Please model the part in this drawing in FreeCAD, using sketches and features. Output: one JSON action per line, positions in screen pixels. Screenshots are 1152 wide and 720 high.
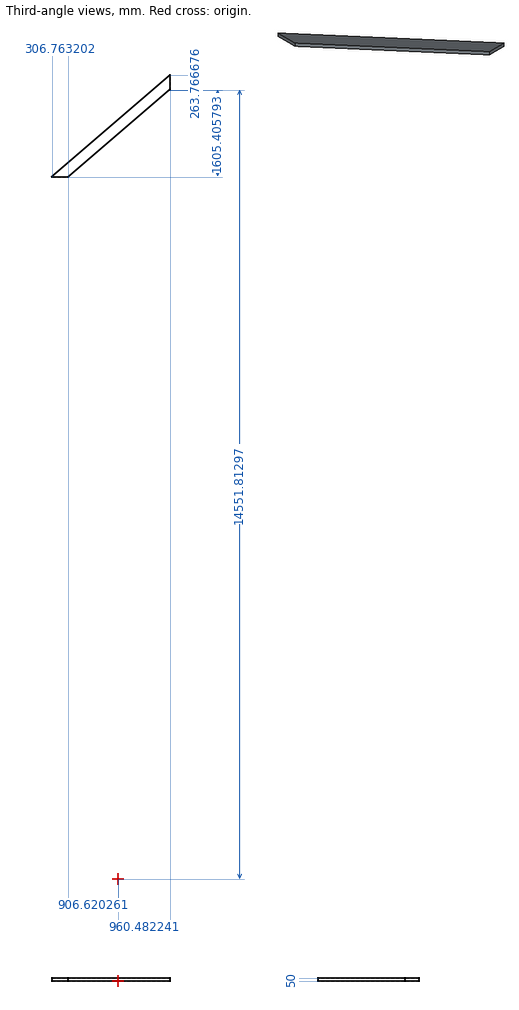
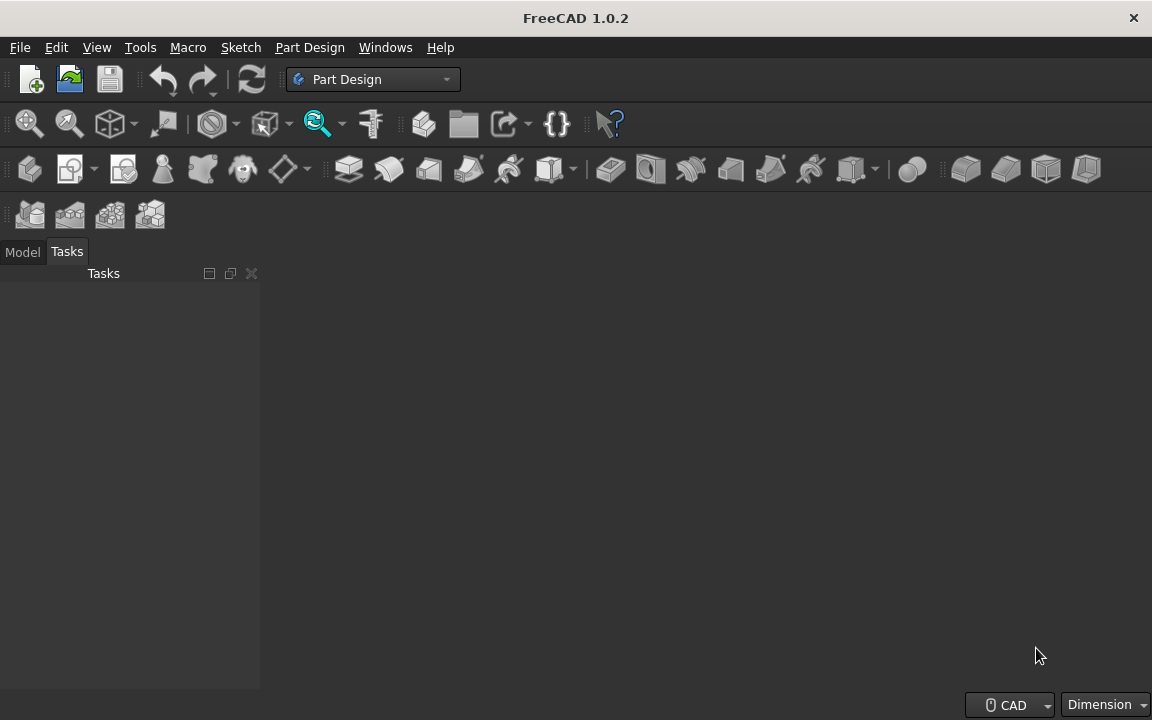
{"action": "key", "text": "ctrl+n"}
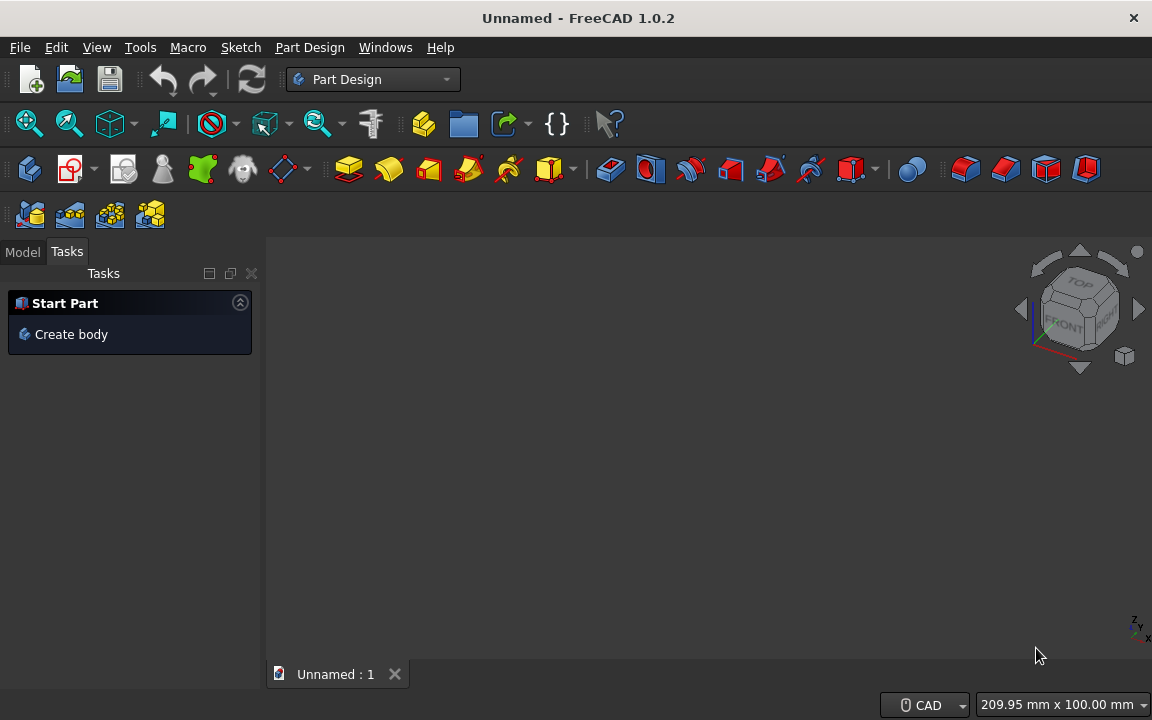
{"action": "left_click", "coordinate": [70, 170]}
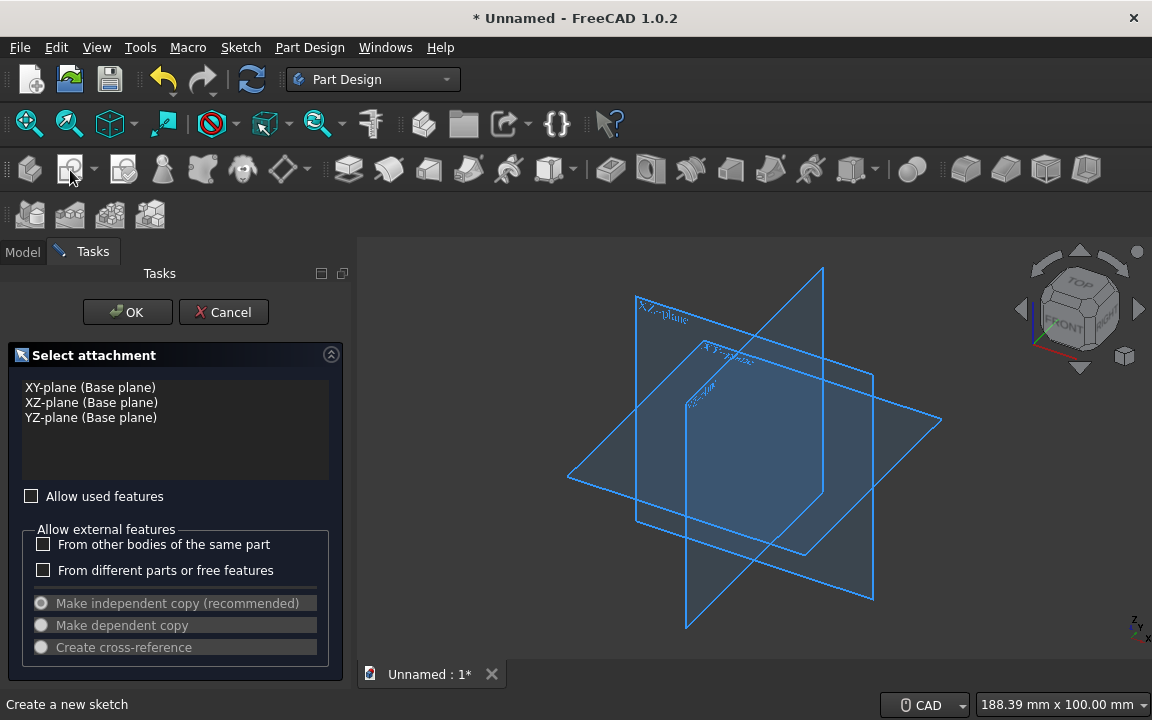
{"action": "left_click", "coordinate": [82, 388]}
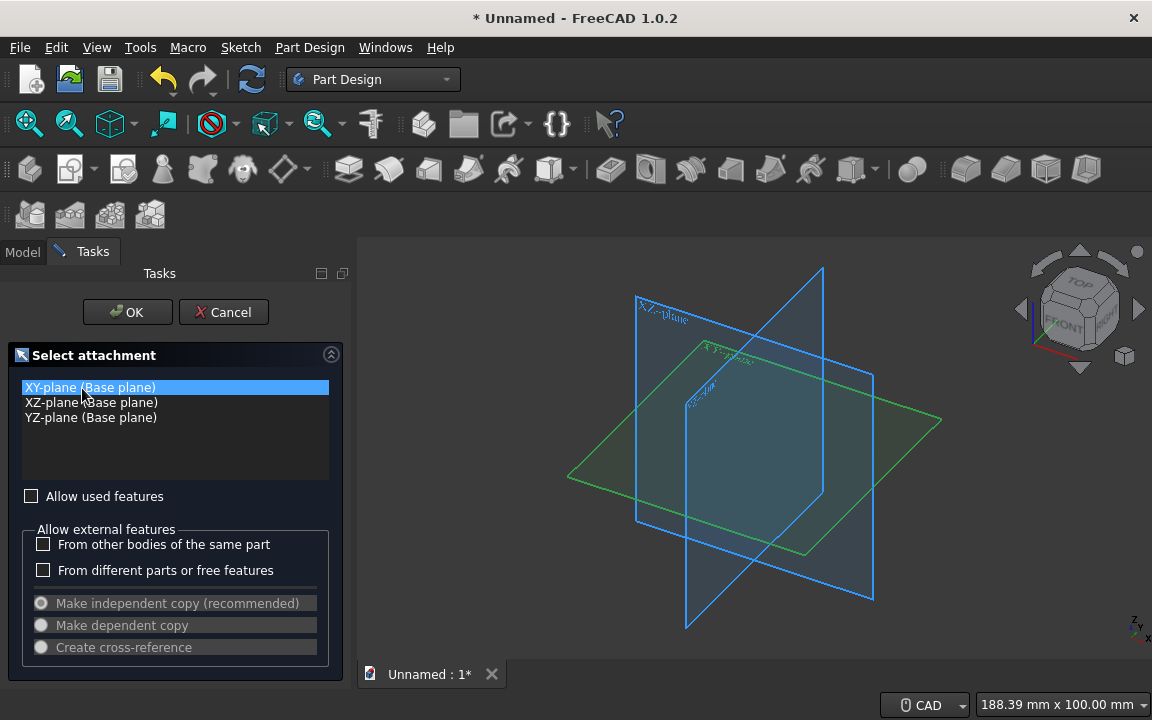
{"action": "left_click", "coordinate": [128, 312]}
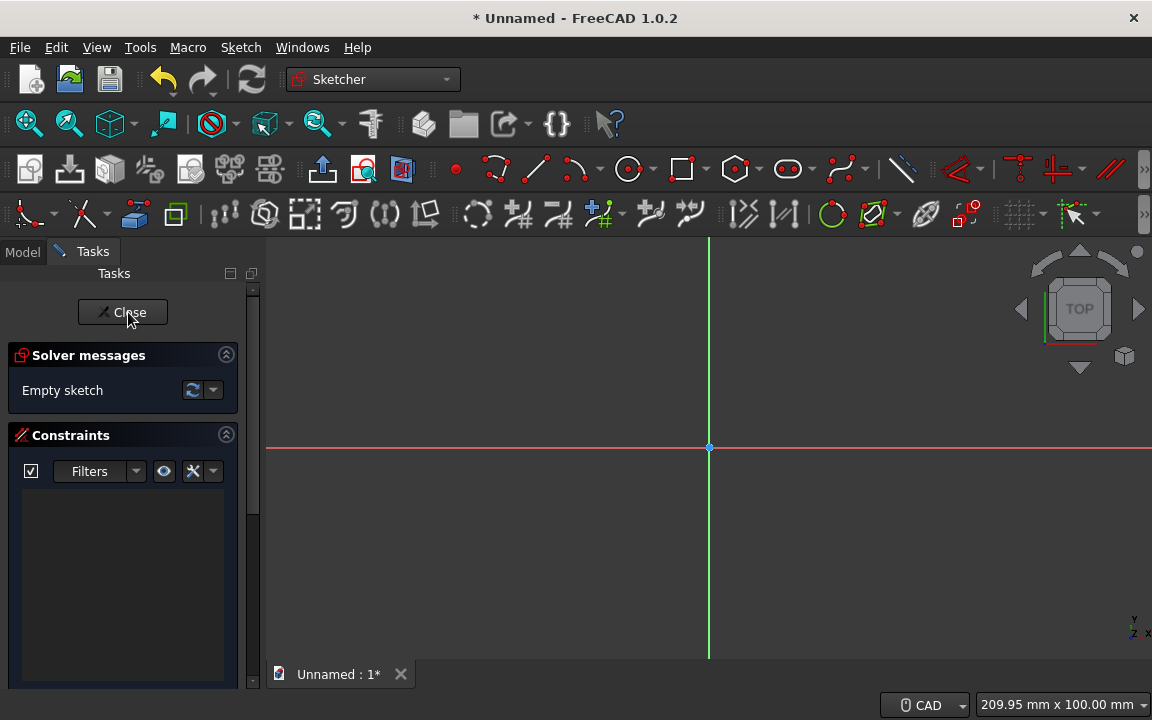
{"action": "scroll", "coordinate": [640, 448], "scroll_direction": "down", "scroll_amount": 15}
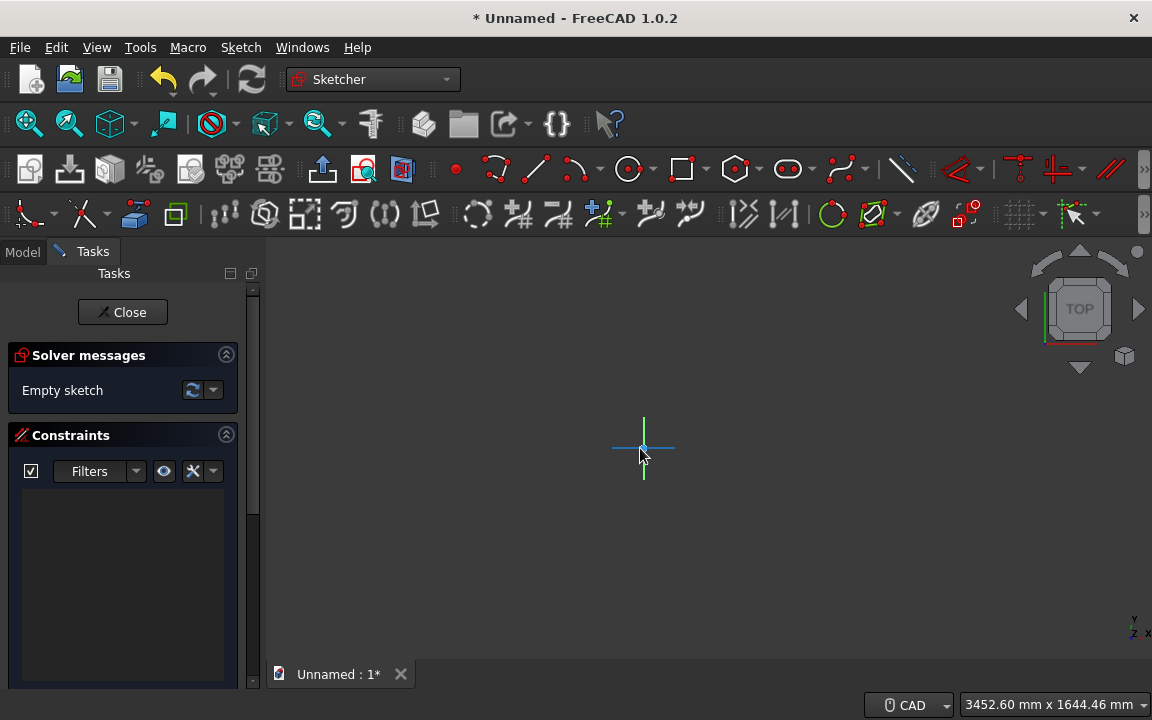
{"action": "scroll", "coordinate": [640, 448], "scroll_direction": "down", "scroll_amount": 5}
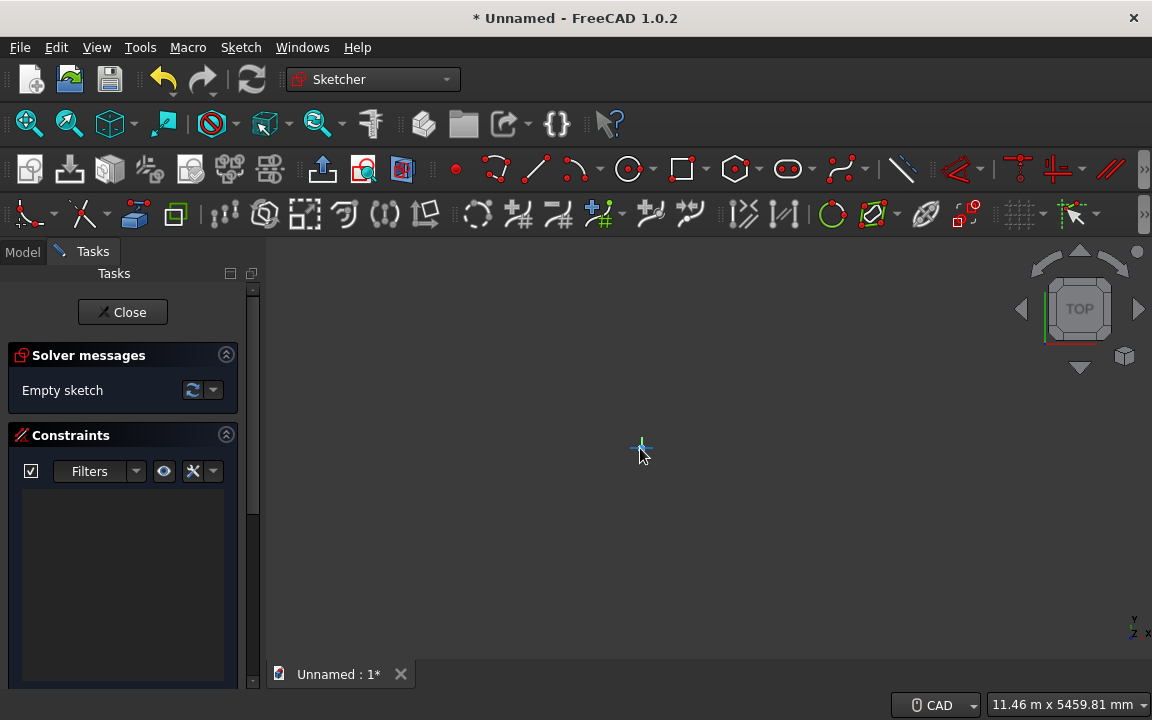
{"action": "scroll", "coordinate": [640, 448], "scroll_direction": "down", "scroll_amount": 5}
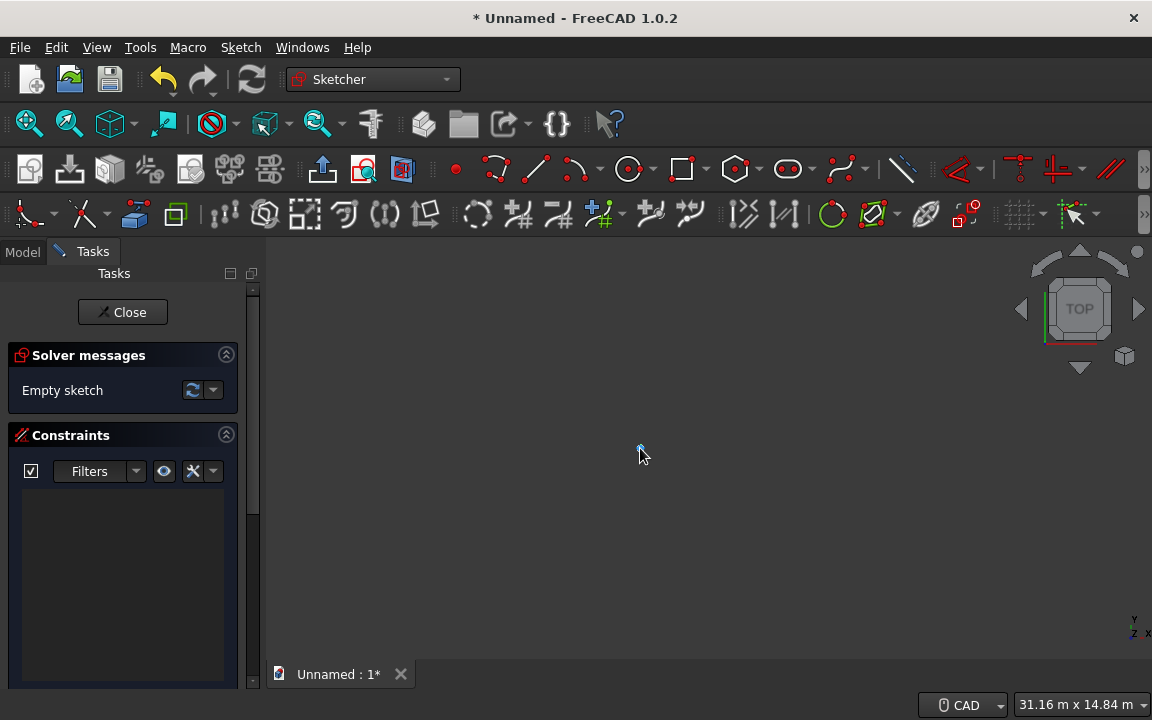
{"action": "scroll", "coordinate": [640, 448], "scroll_direction": "down", "scroll_amount": 5}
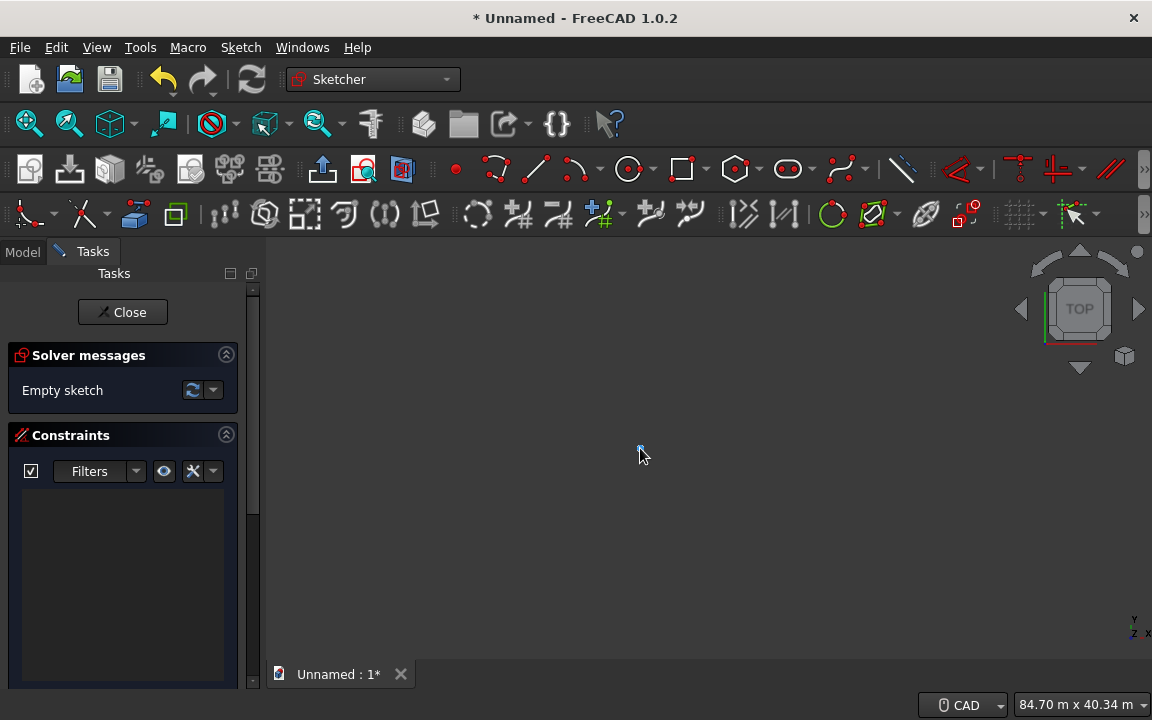
{"action": "scroll", "coordinate": [639, 292], "scroll_direction": "up", "scroll_amount": 13}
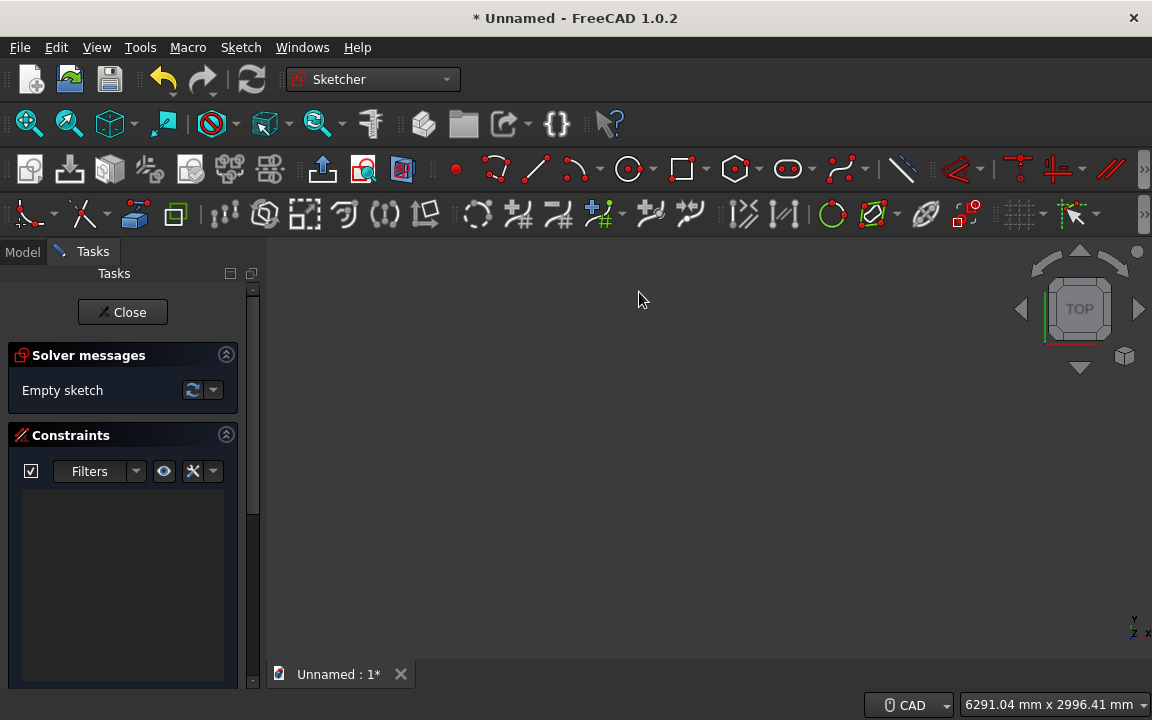
{"action": "key", "text": "g m"}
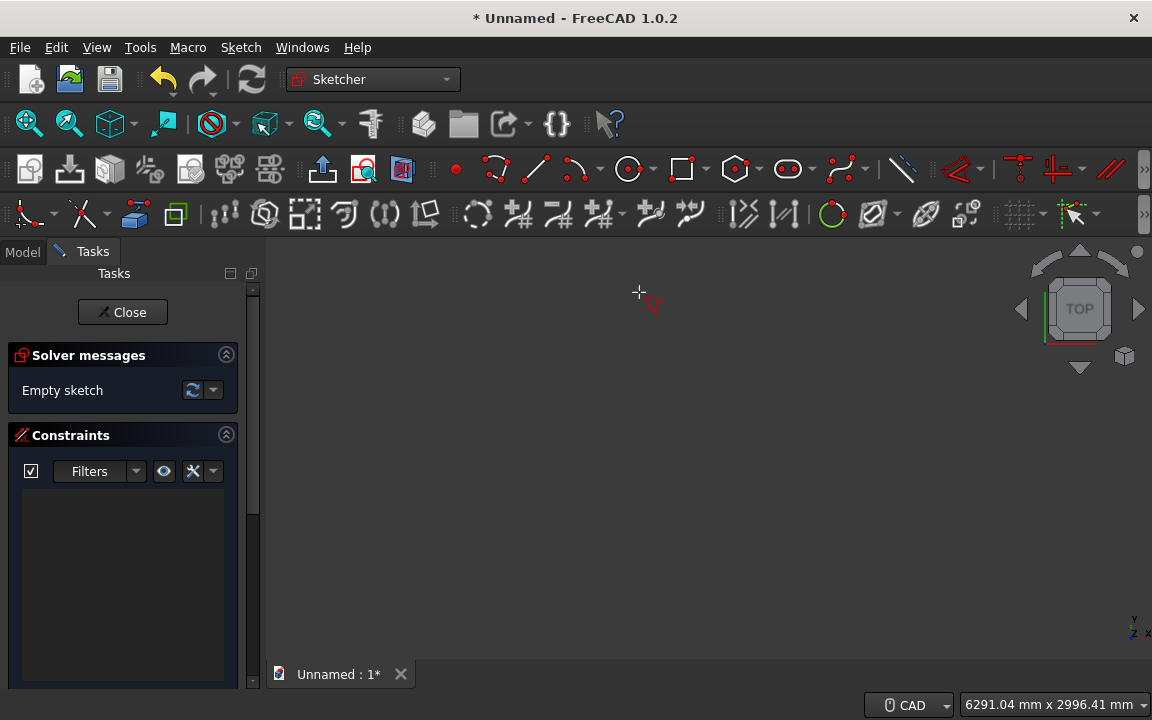
{"action": "left_click", "coordinate": [528, 574]}
{"action": "left_click", "coordinate": [790, 348]}
{"action": "left_click", "coordinate": [790, 311]}
{"action": "left_click", "coordinate": [484, 574]}
{"action": "left_click", "coordinate": [528, 575]}
{"action": "key", "text": "Escape"}
{"action": "key", "text": "Escape"}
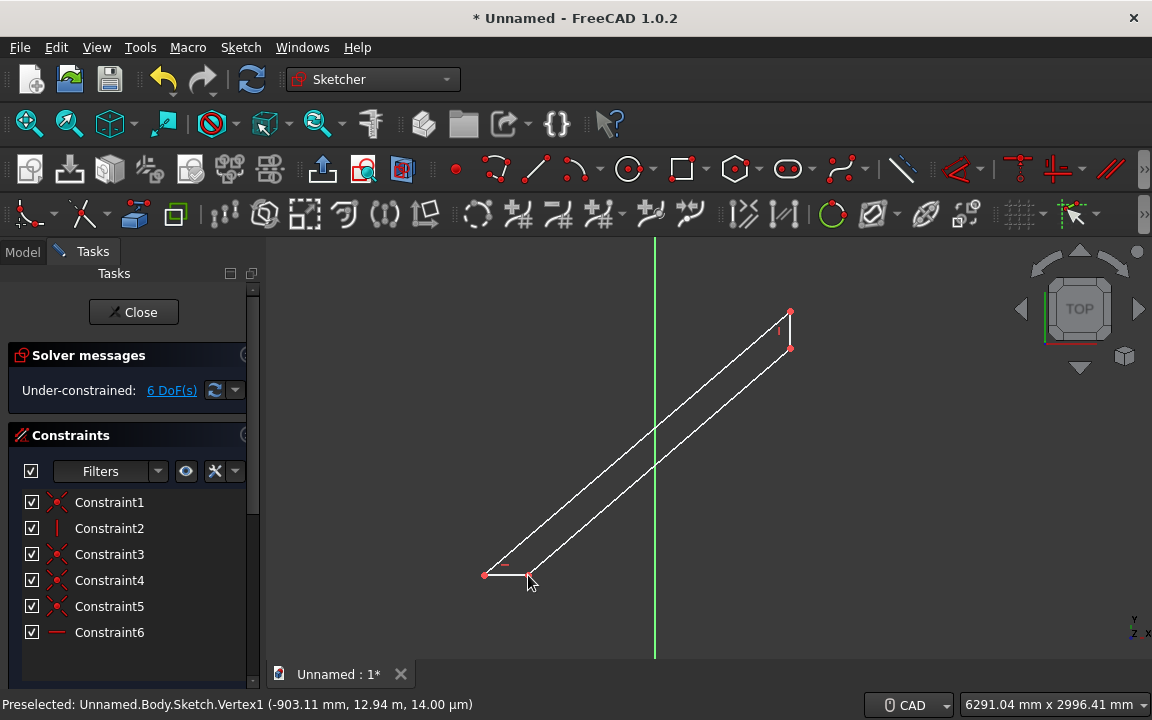
{"action": "key", "text": "d"}